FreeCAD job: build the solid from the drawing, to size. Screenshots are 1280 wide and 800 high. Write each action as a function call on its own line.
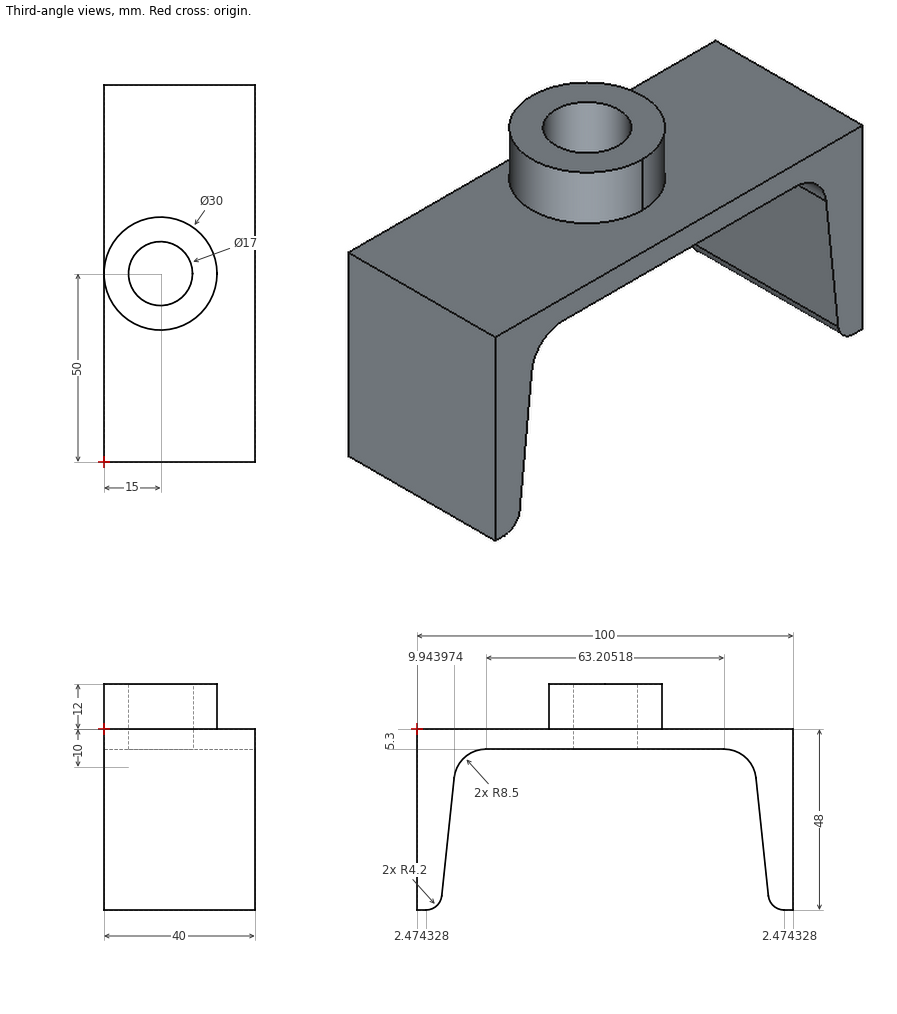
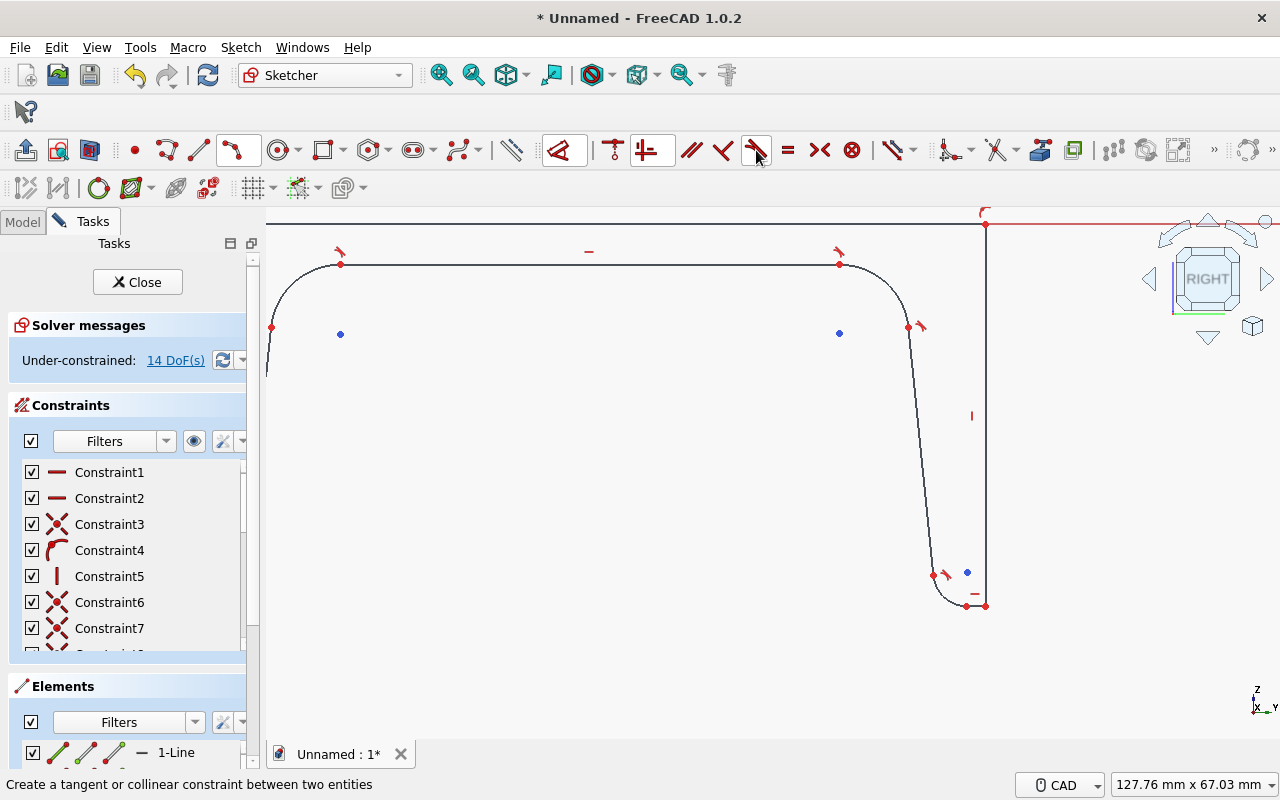
scroll(976, 606, up, 2)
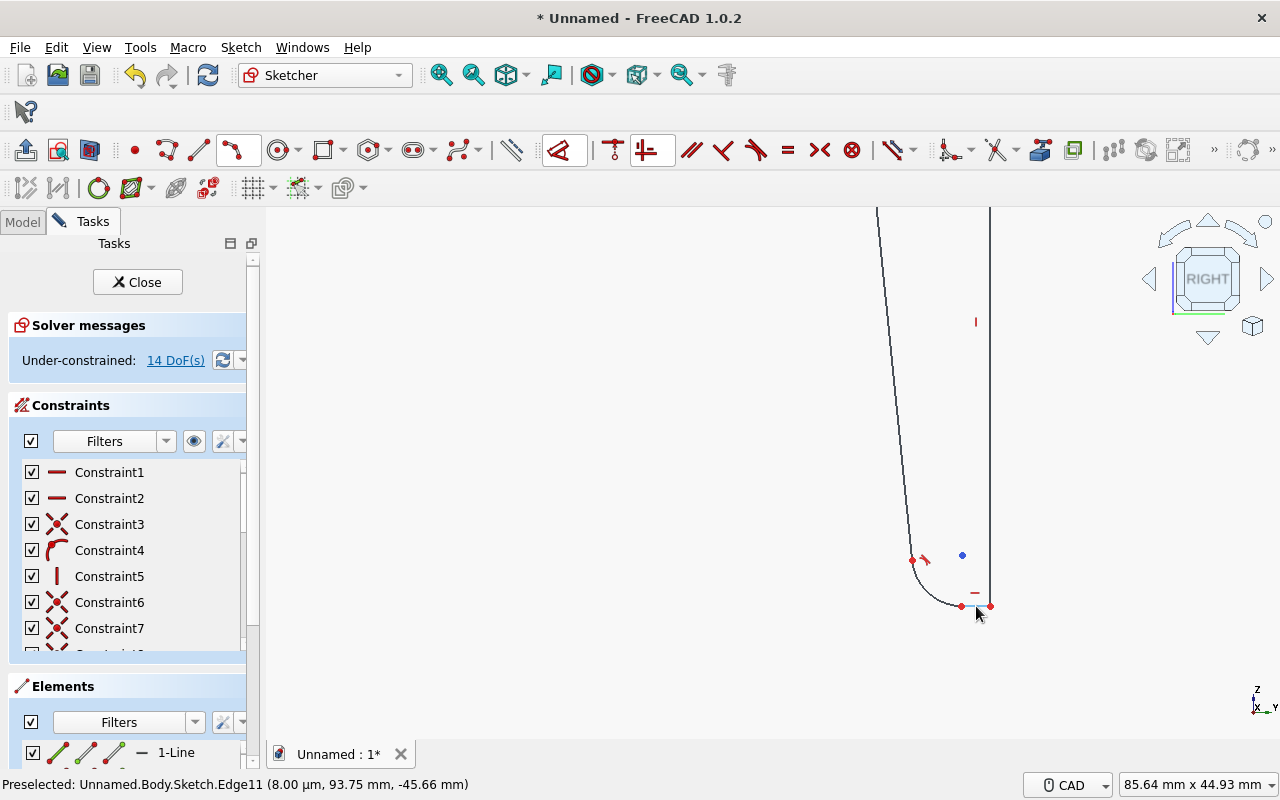
click(976, 606)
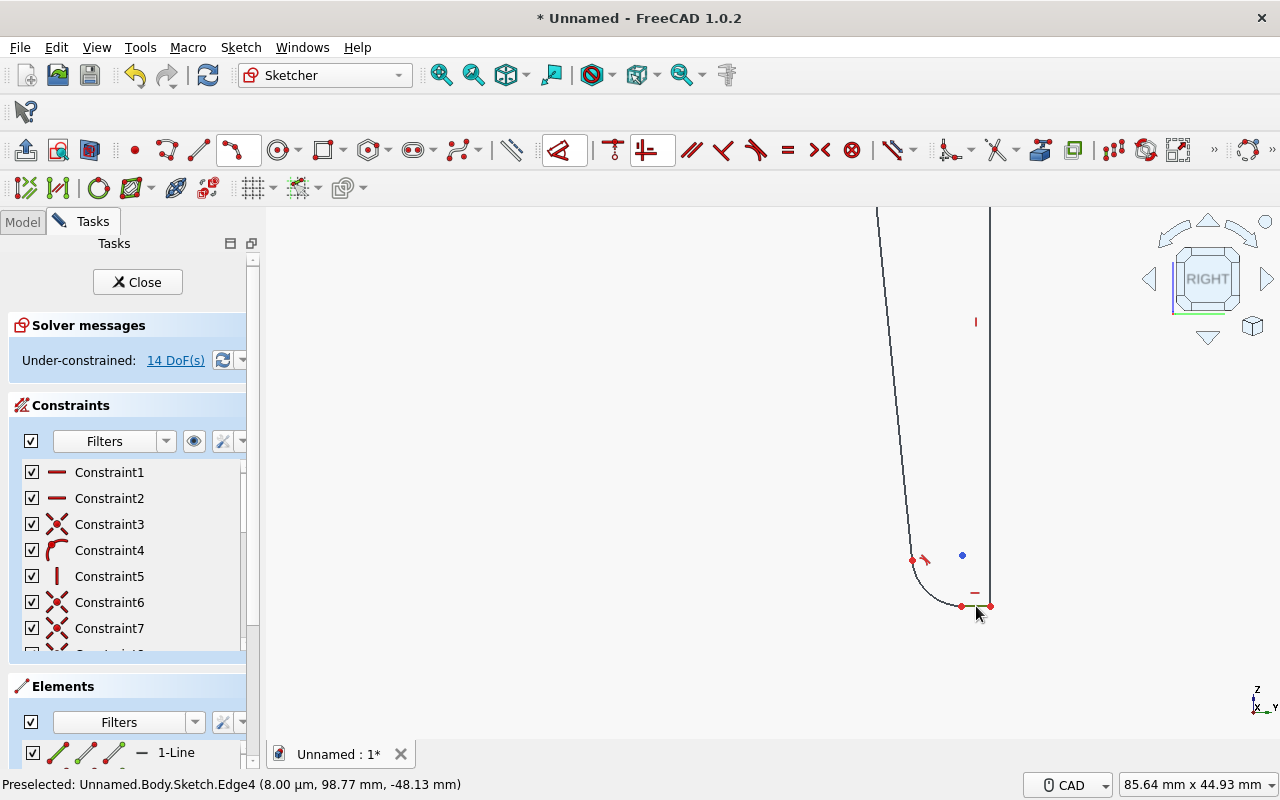
click(919, 581)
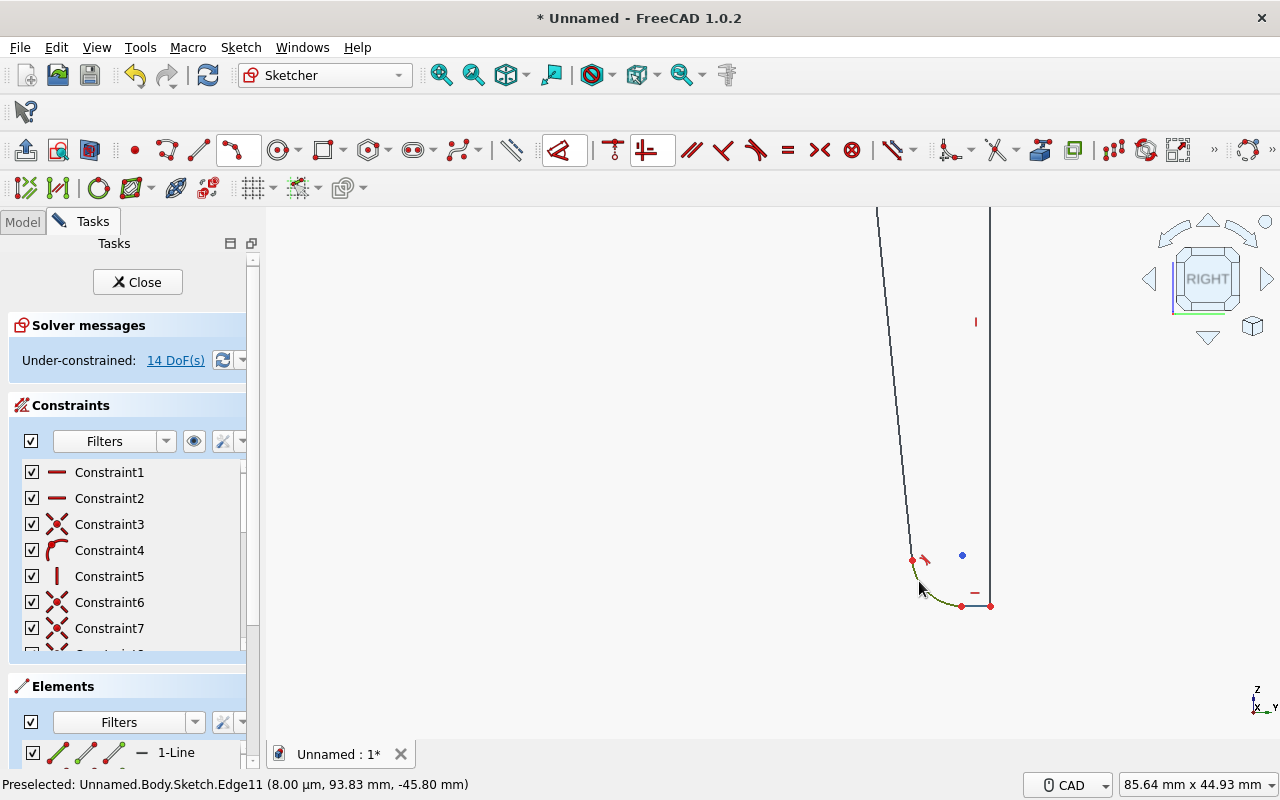
click(756, 150)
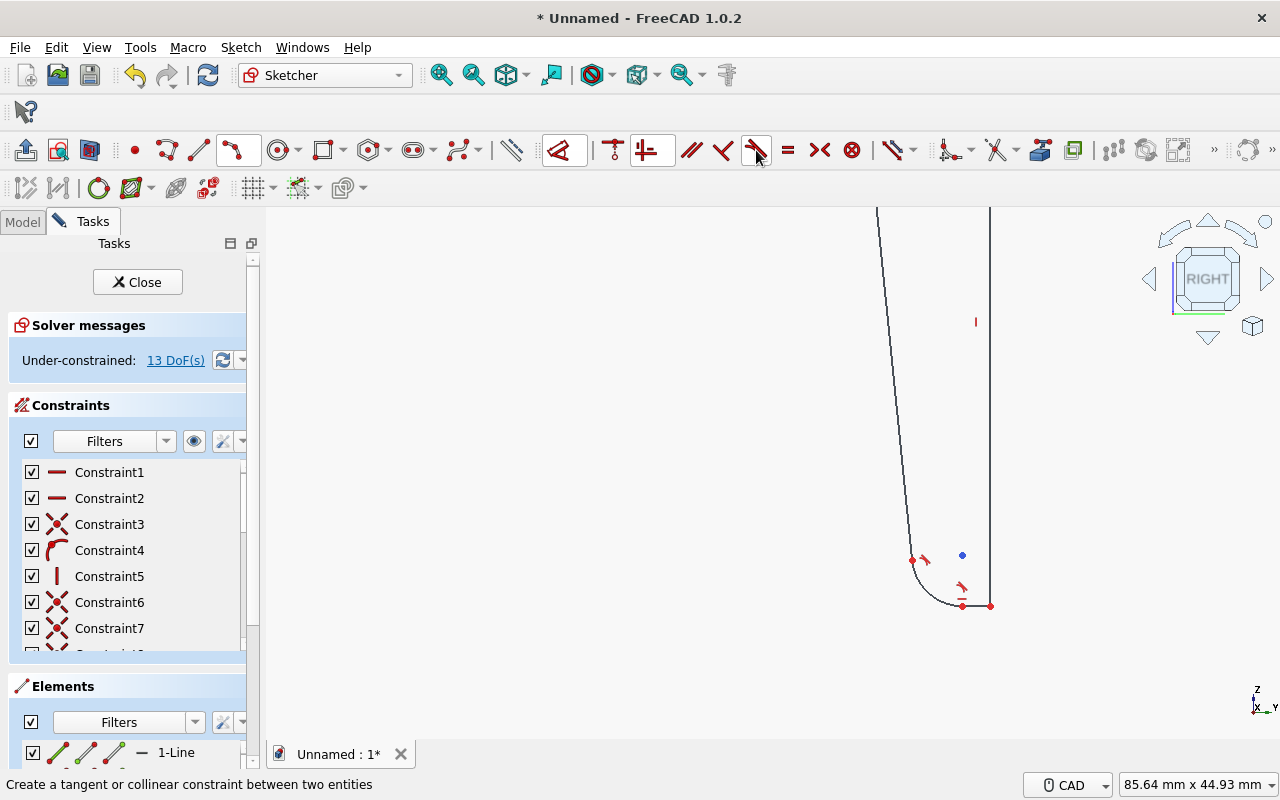
scroll(954, 597, down, 4)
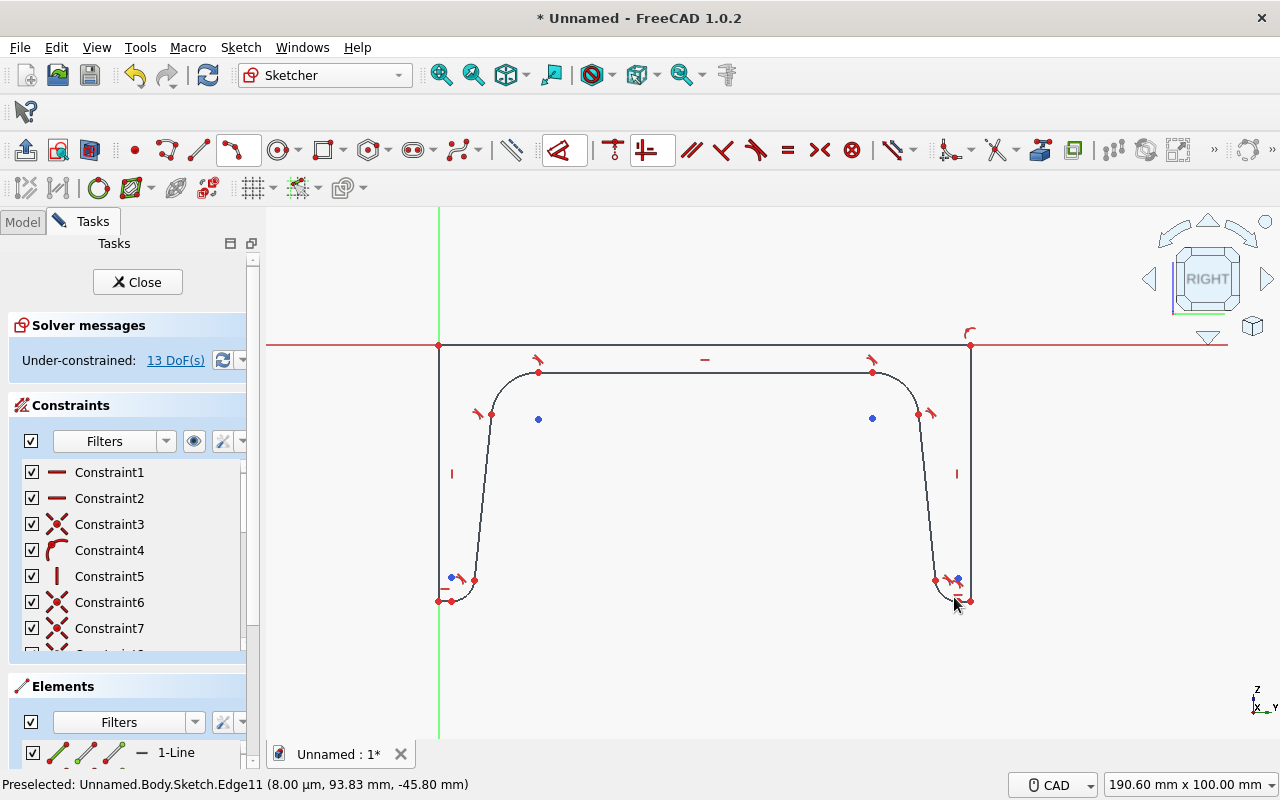
scroll(444, 601, up, 5)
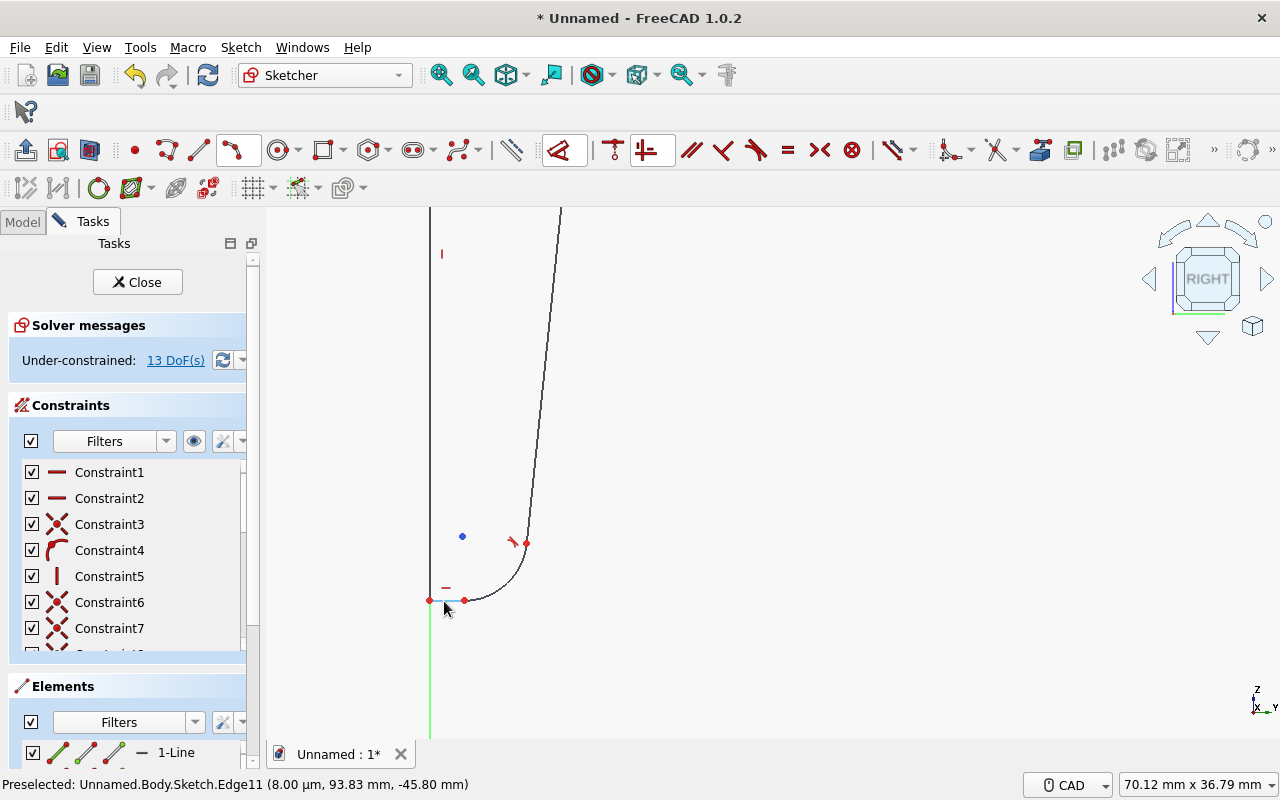
click(443, 601)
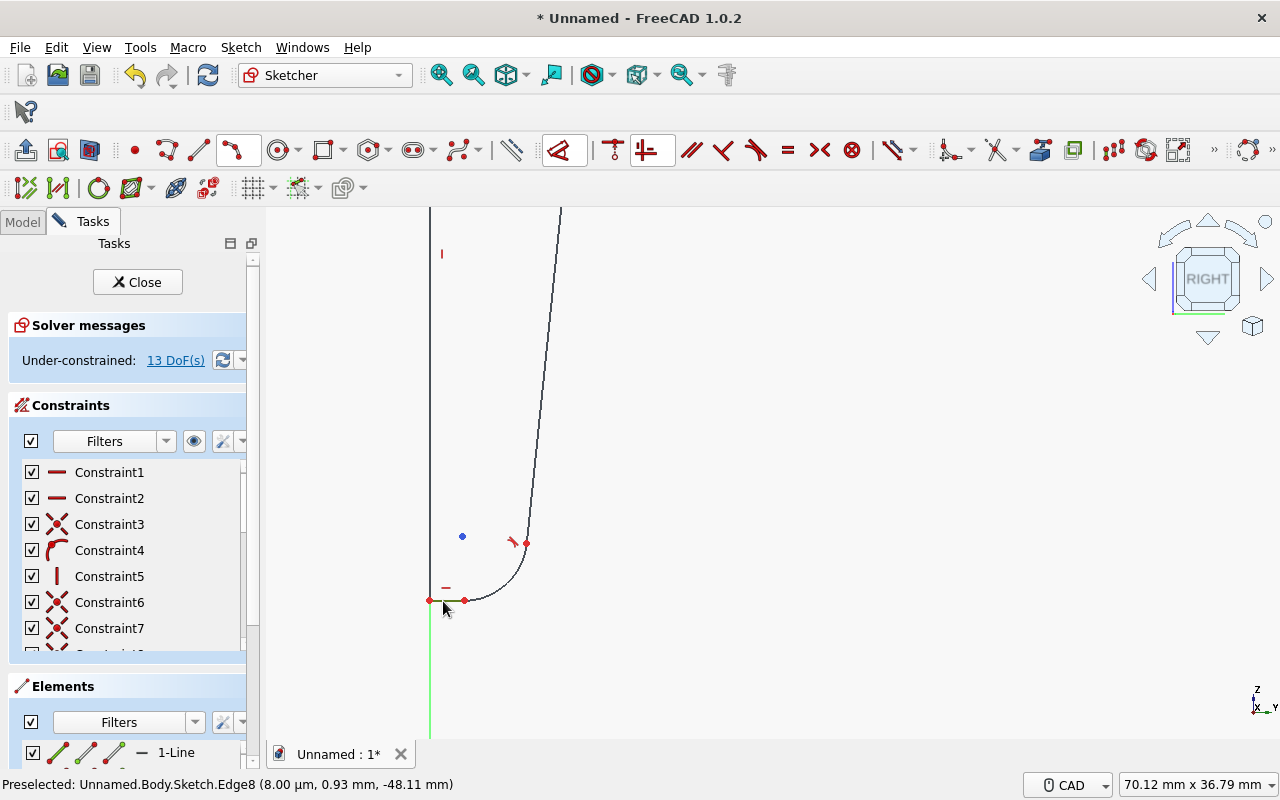
click(491, 594)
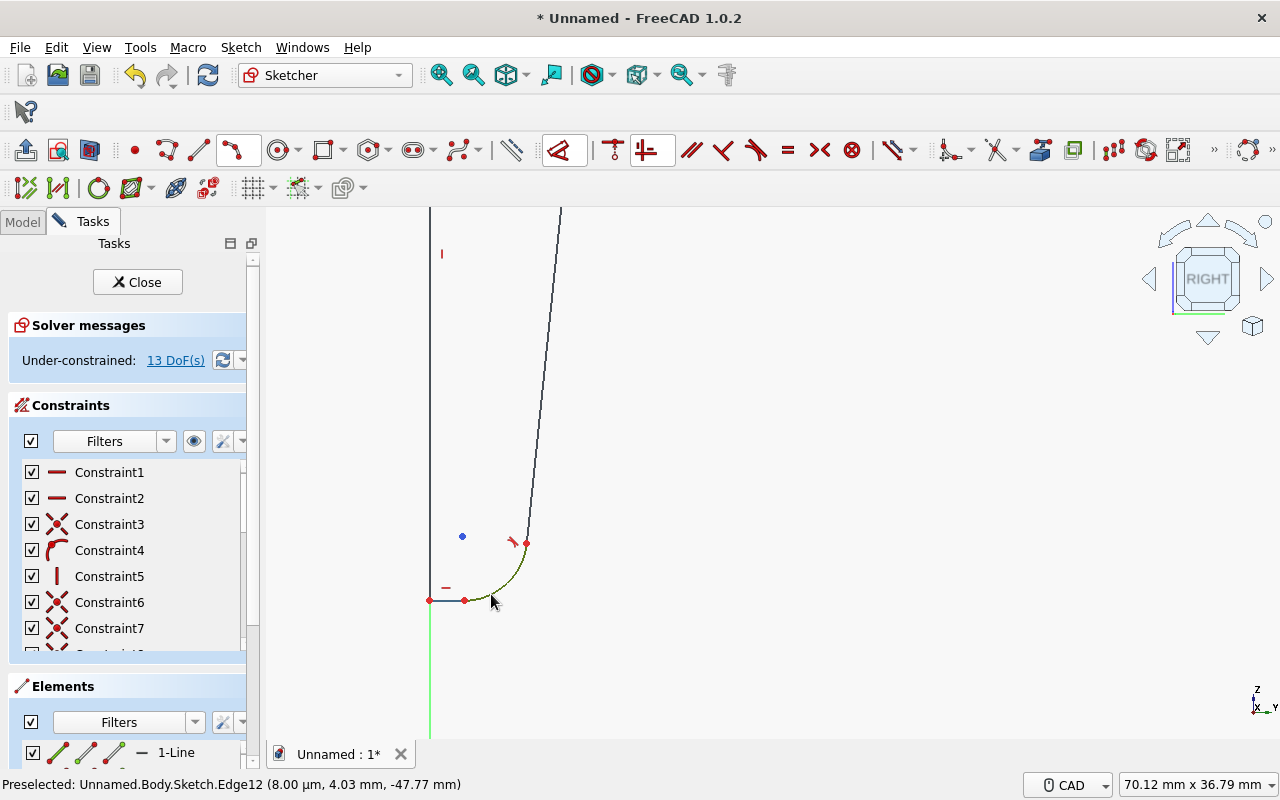
click(756, 150)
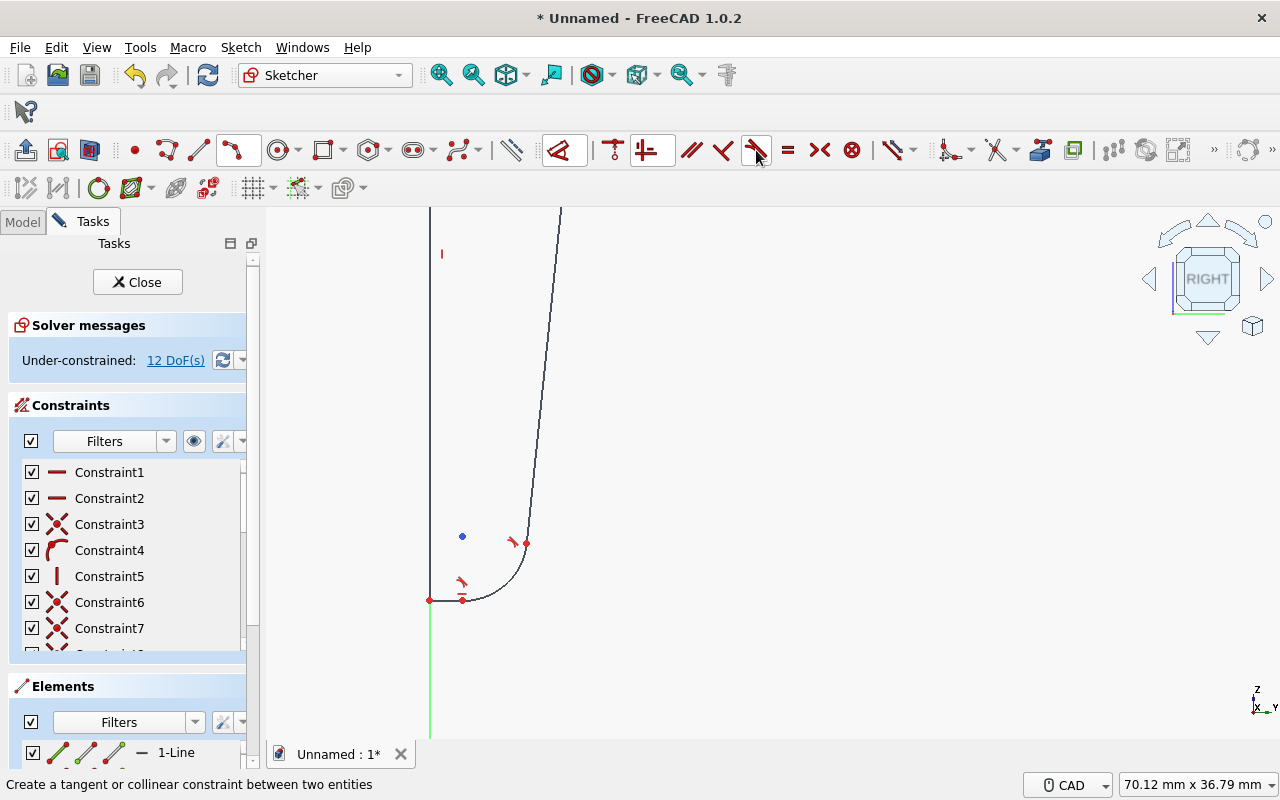
scroll(444, 601, down, 5)